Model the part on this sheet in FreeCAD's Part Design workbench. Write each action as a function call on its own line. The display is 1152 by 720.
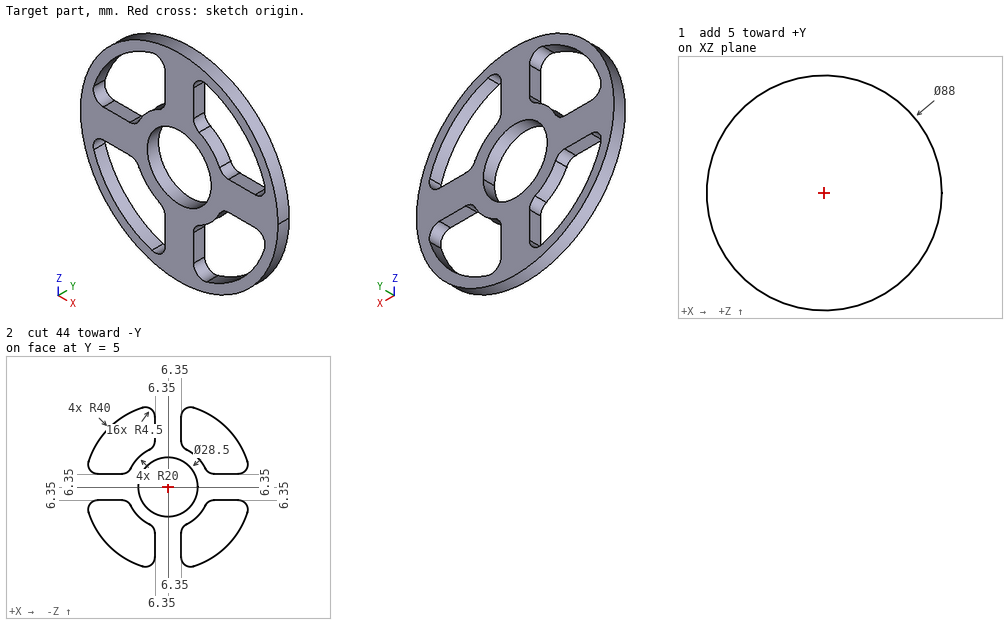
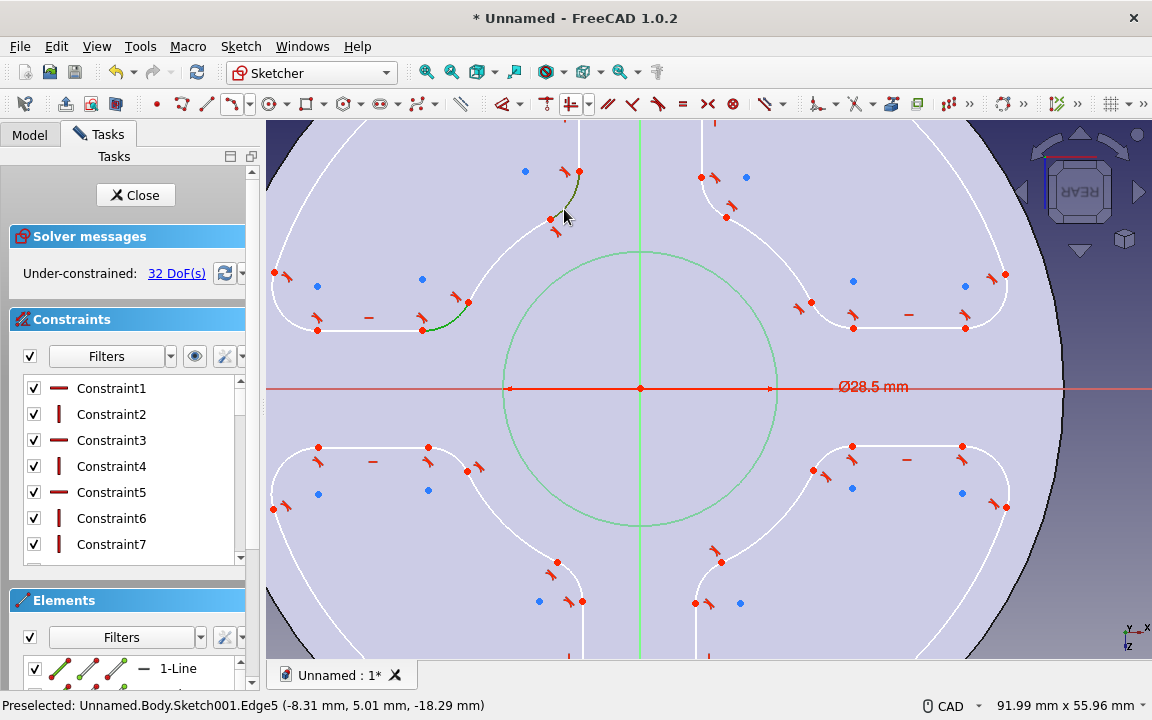
scroll(641, 390, down, 4)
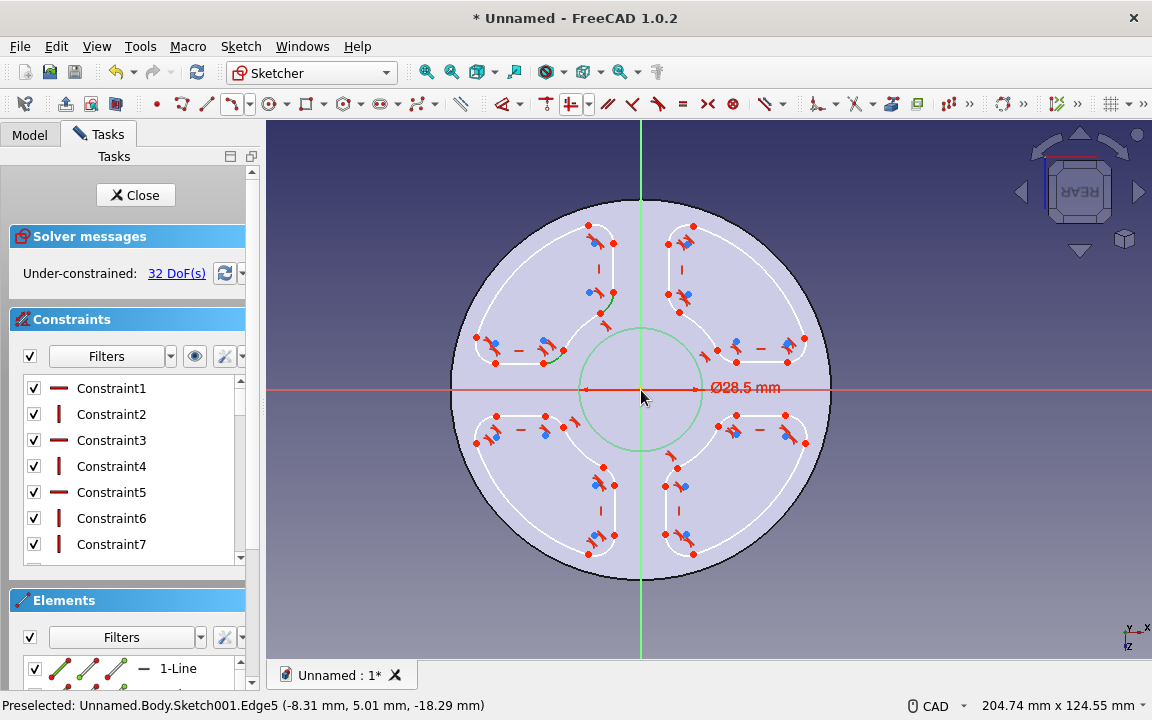
scroll(610, 233, up, 2)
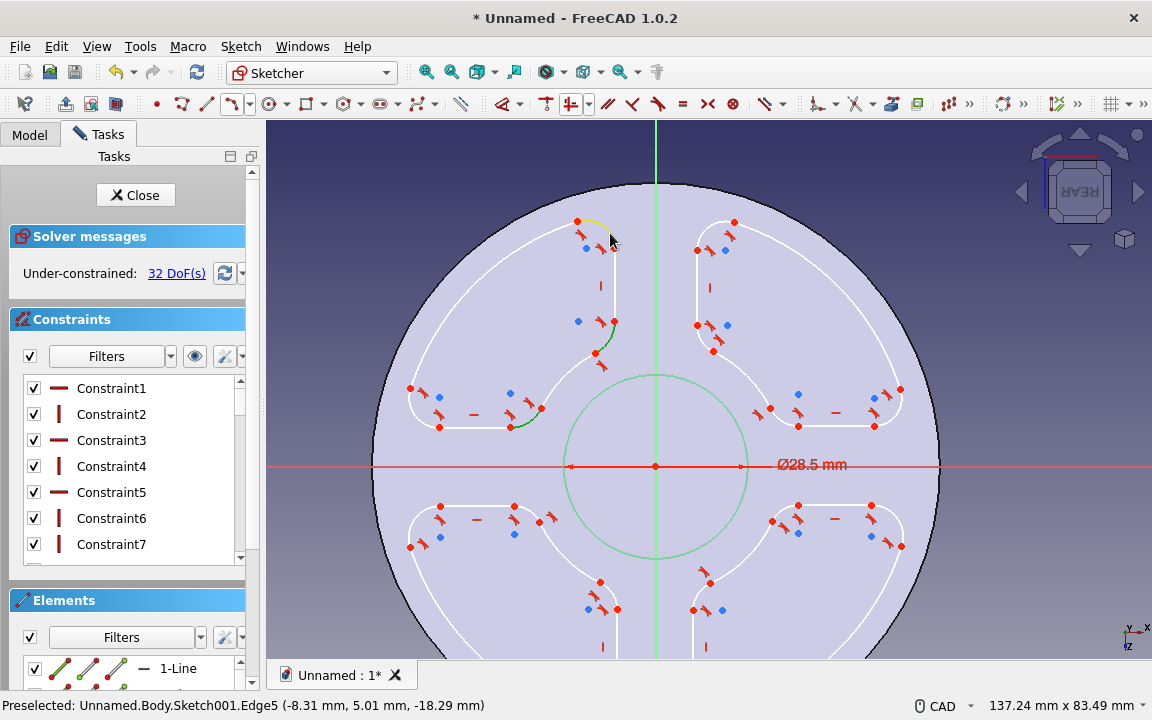
click(610, 234)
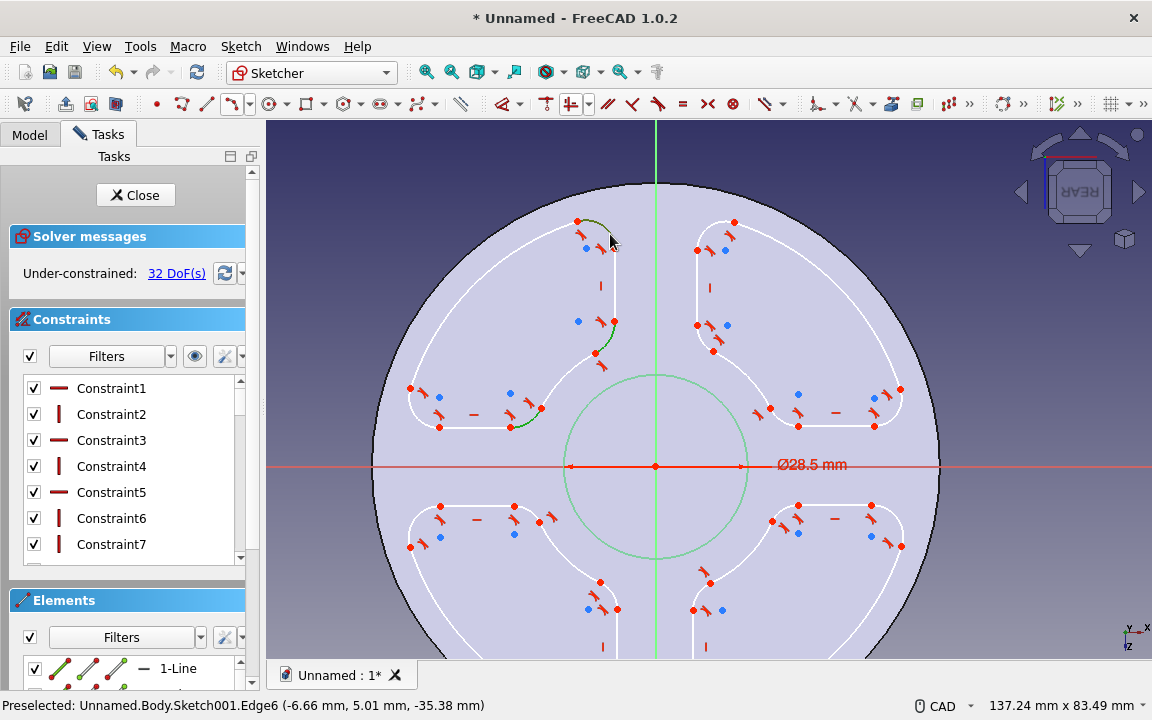
click(410, 405)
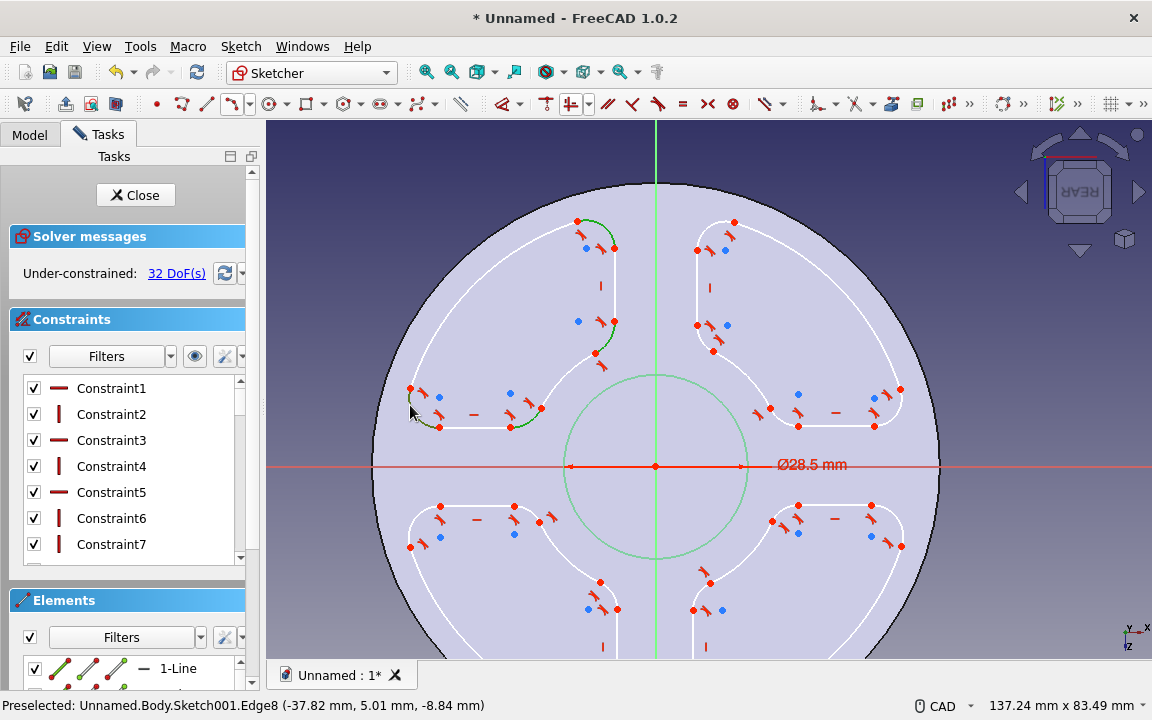
click(889, 422)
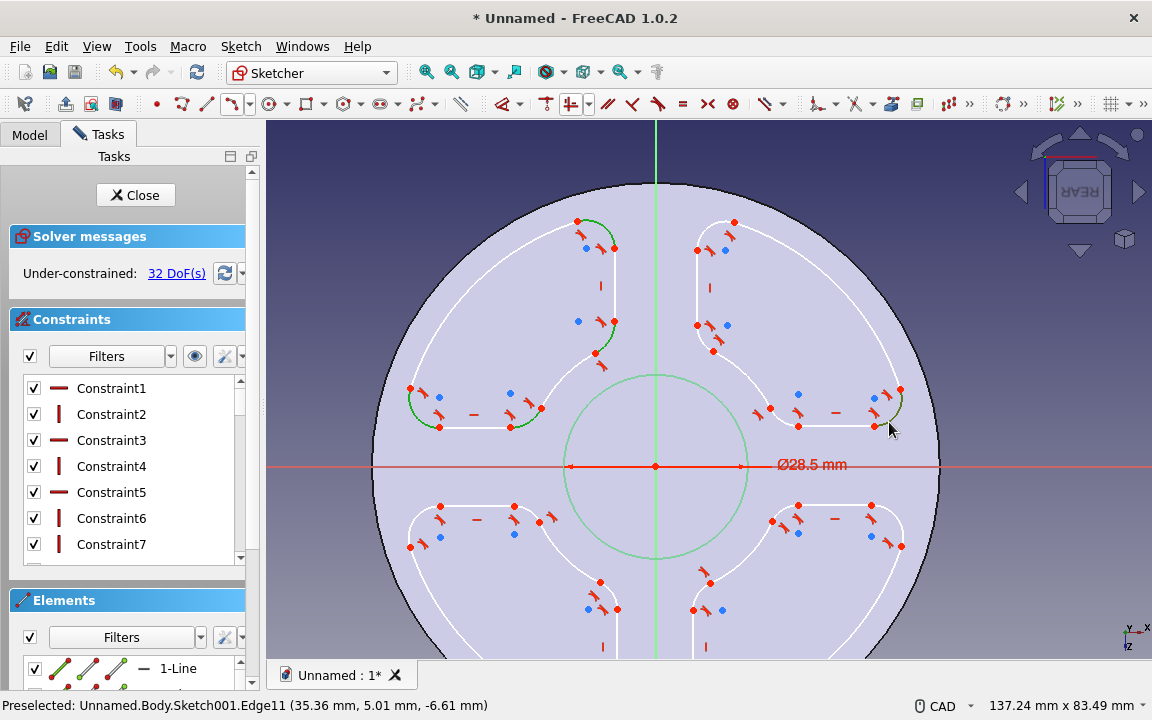
click(719, 222)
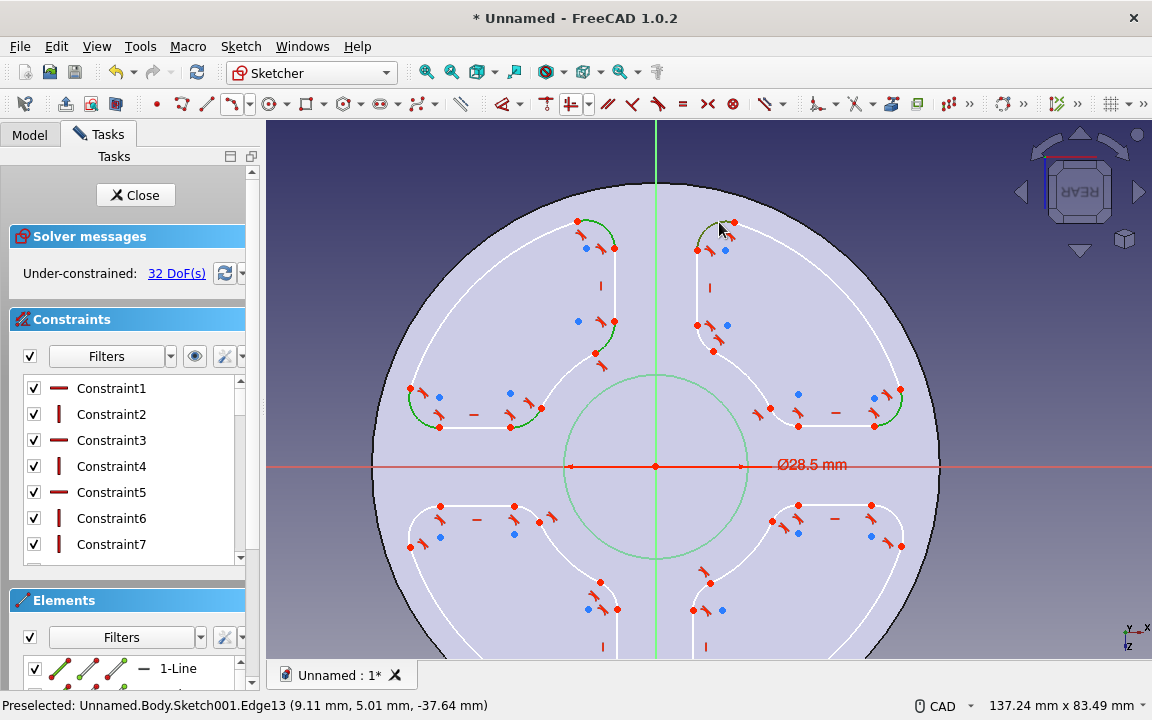
scroll(699, 335, up, 2)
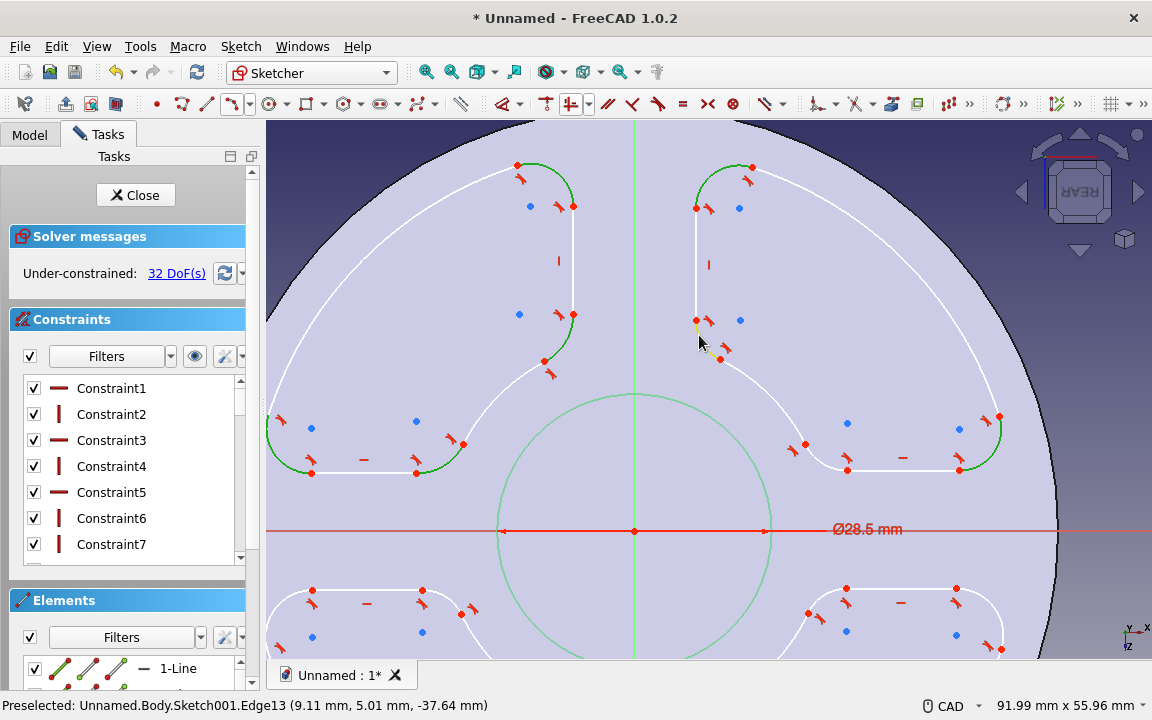
click(698, 335)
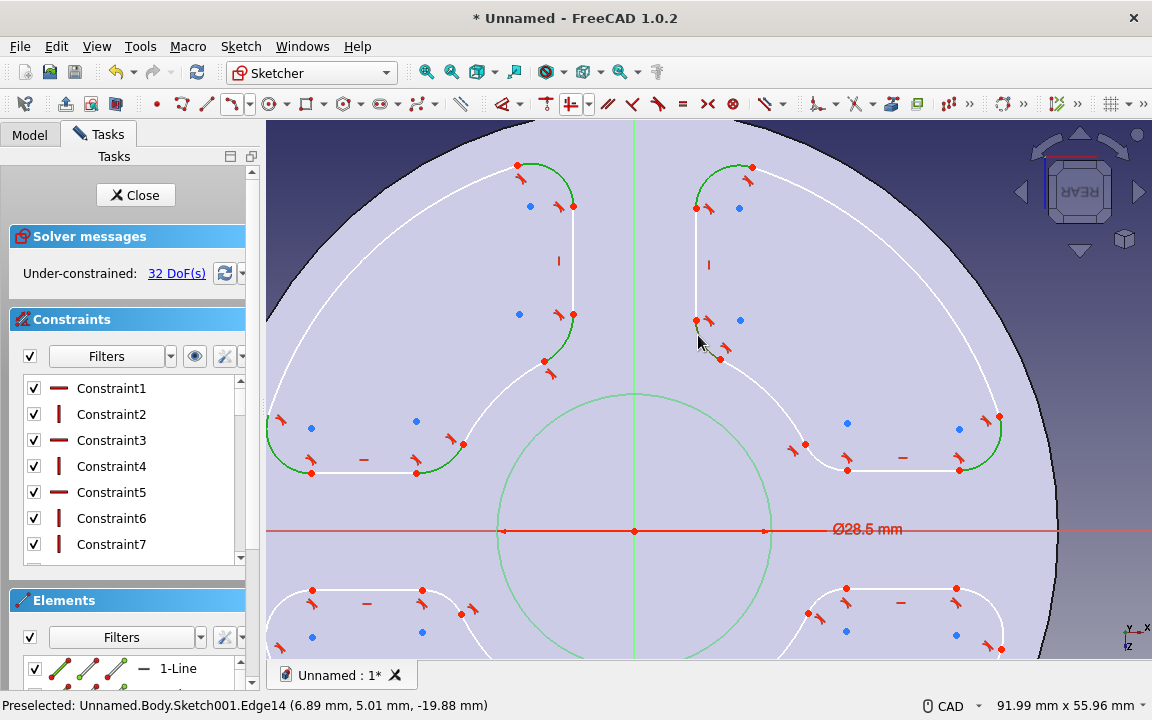
click(815, 457)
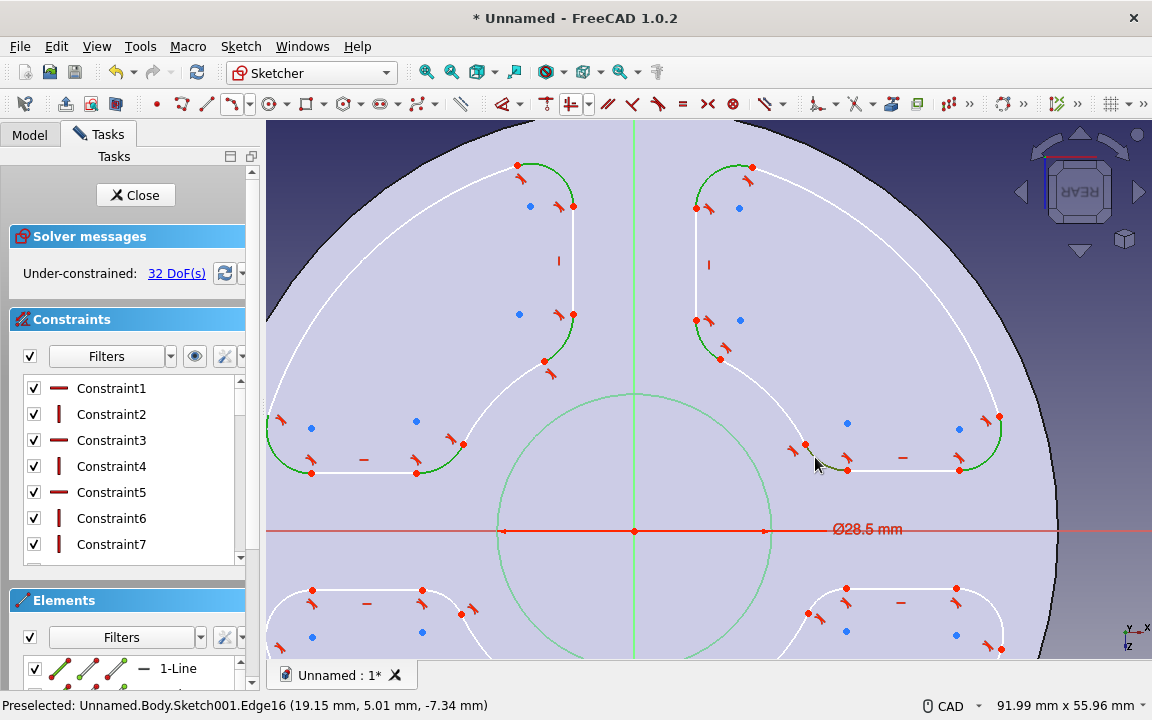
click(833, 591)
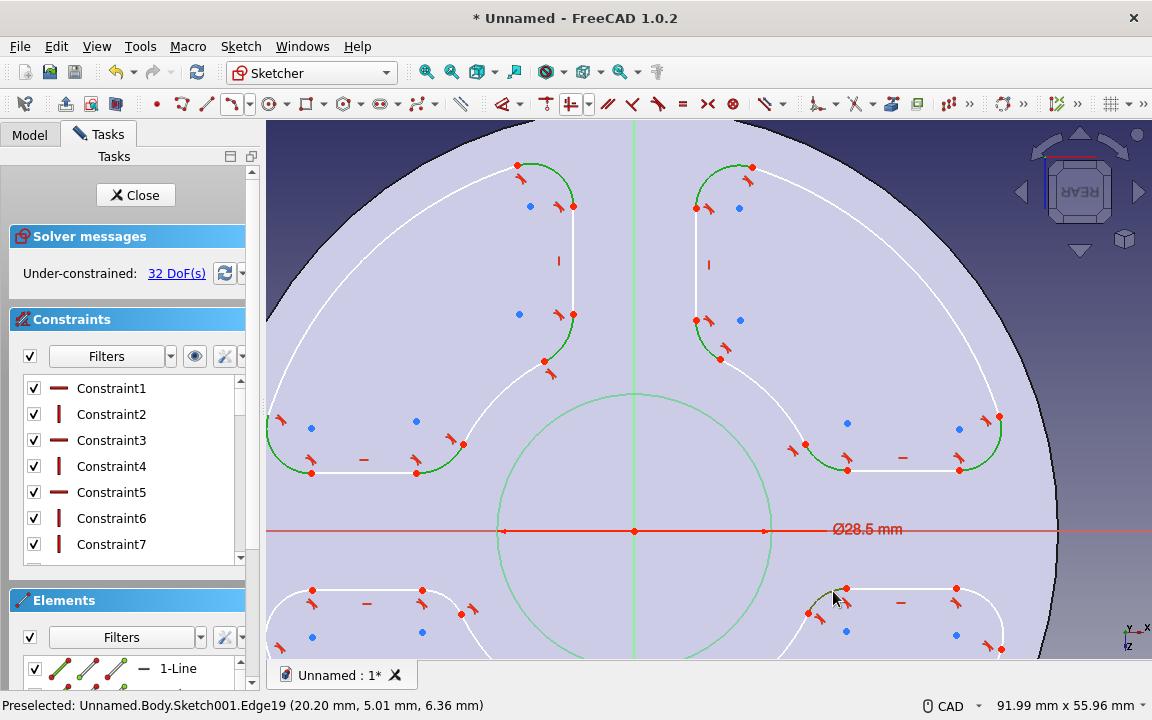
scroll(645, 274, down, 4)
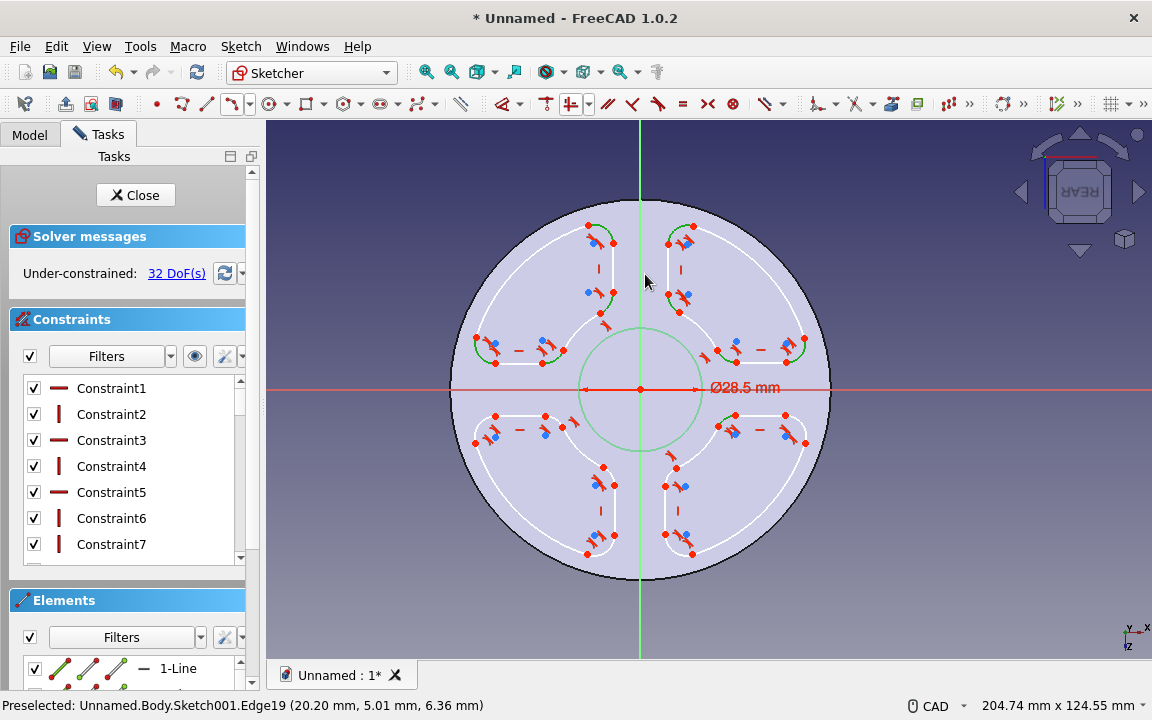
scroll(671, 472, up, 4)